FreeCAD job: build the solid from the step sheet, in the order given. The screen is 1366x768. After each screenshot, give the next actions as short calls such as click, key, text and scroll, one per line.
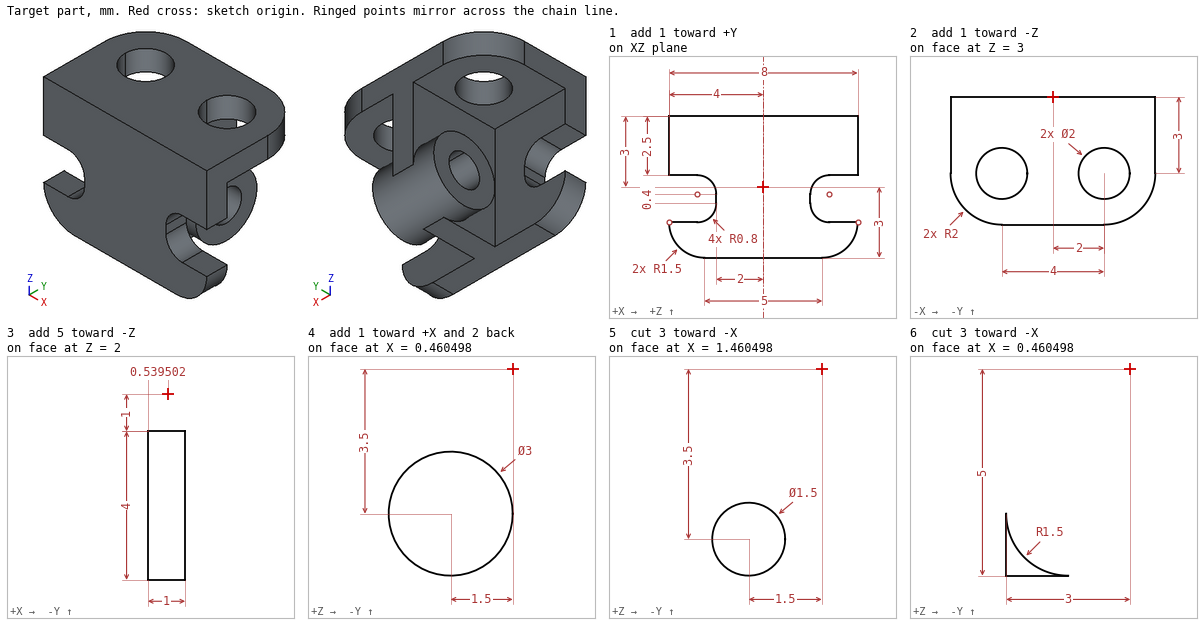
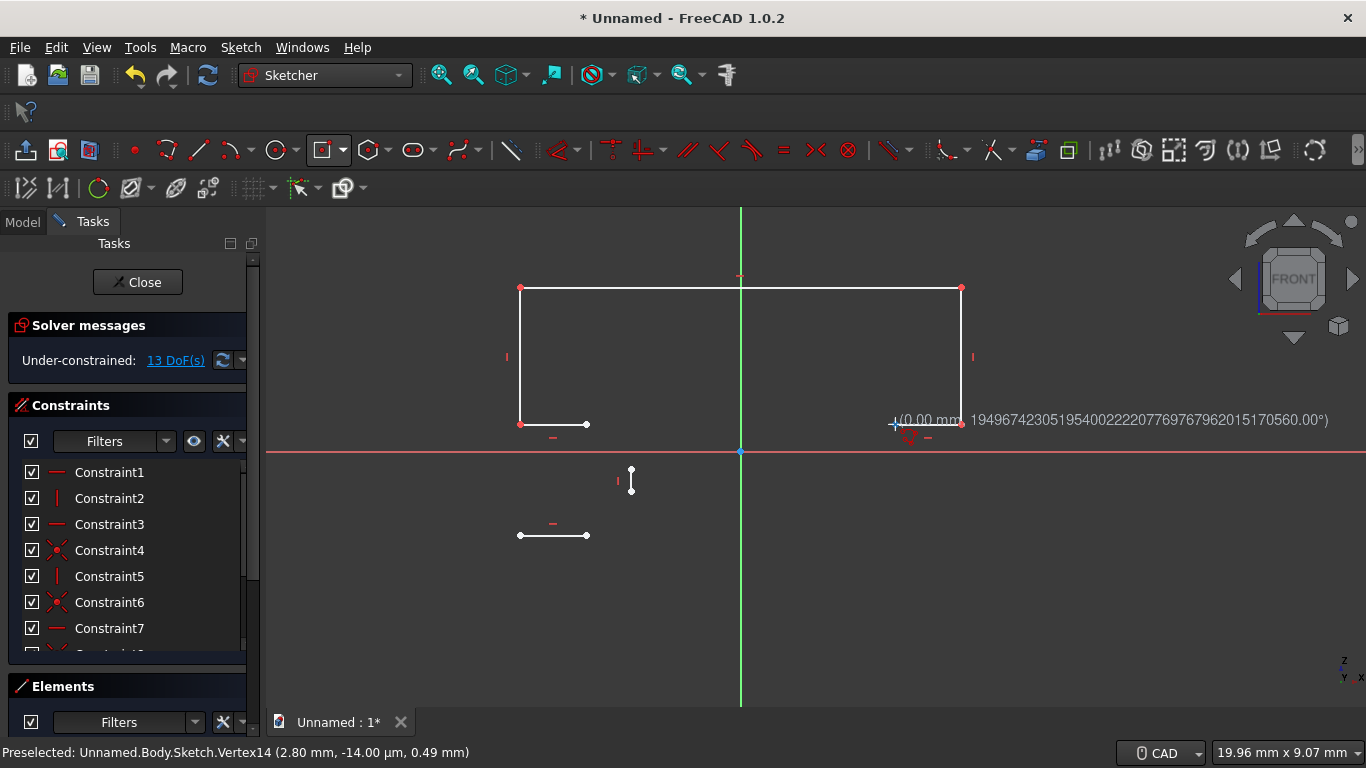
click(200, 150)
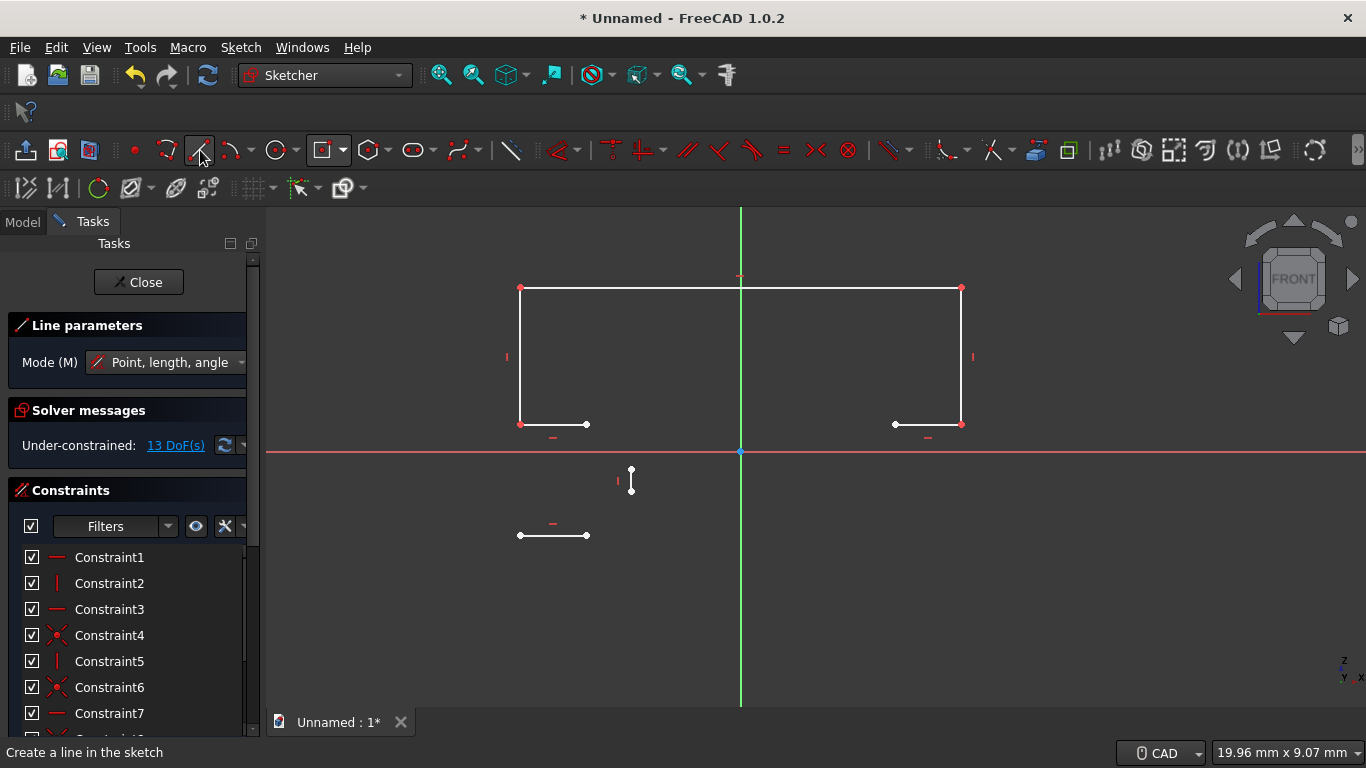
click(851, 469)
click(851, 491)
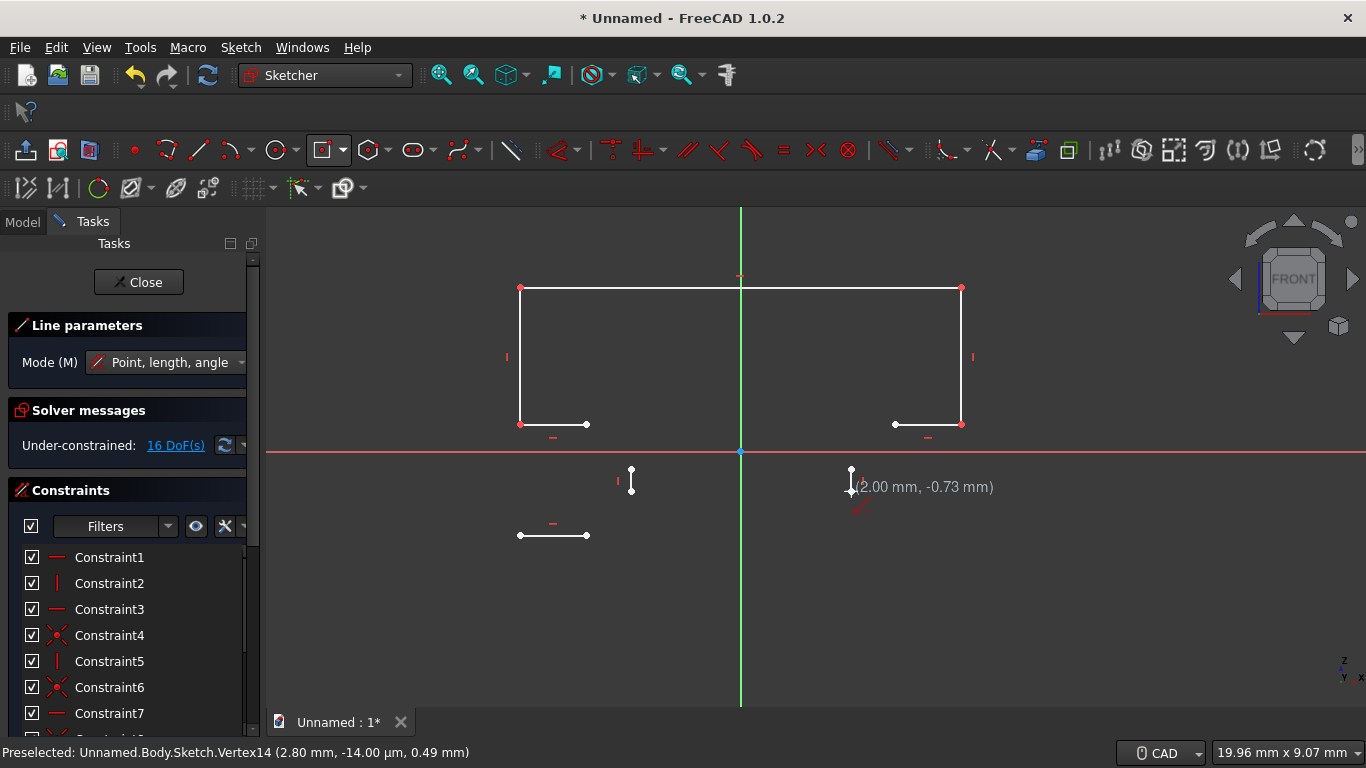
click(895, 535)
click(961, 535)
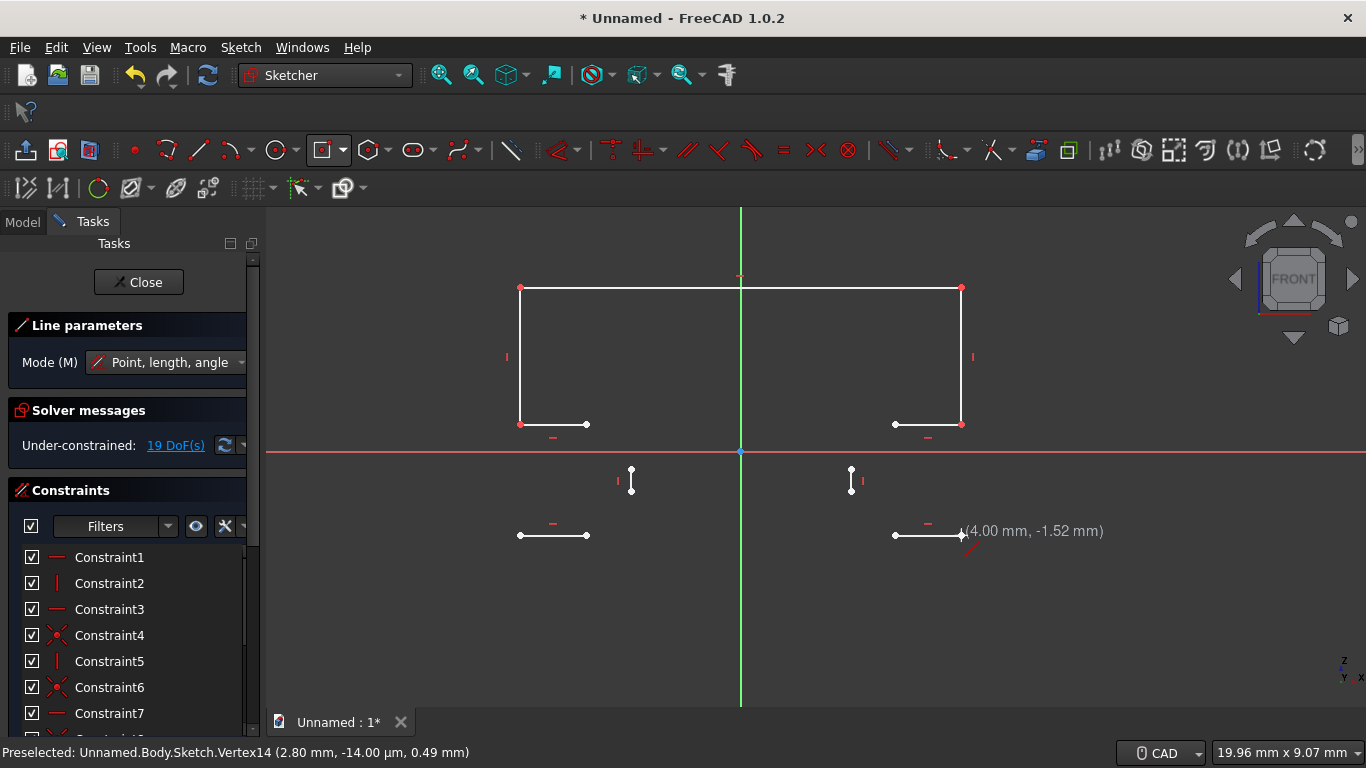
click(879, 617)
click(603, 617)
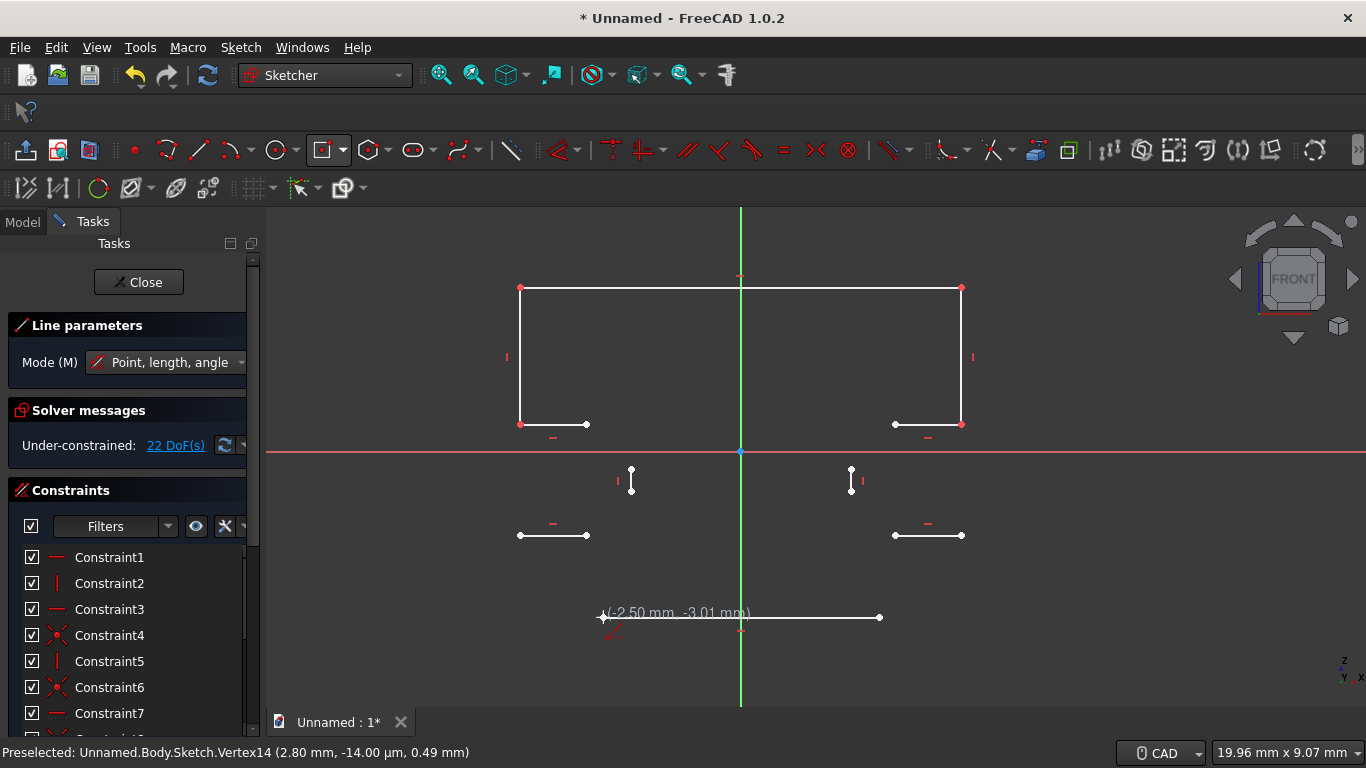
click(254, 150)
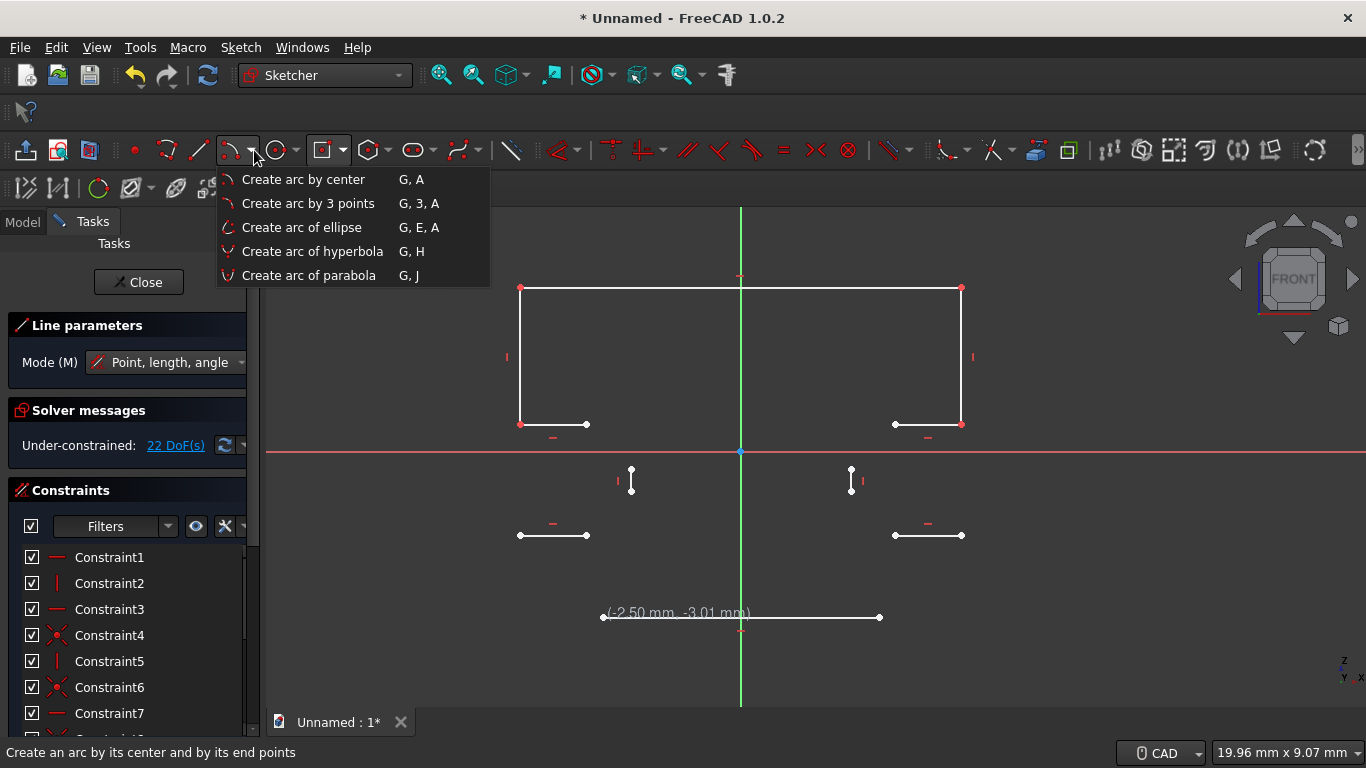
click(354, 203)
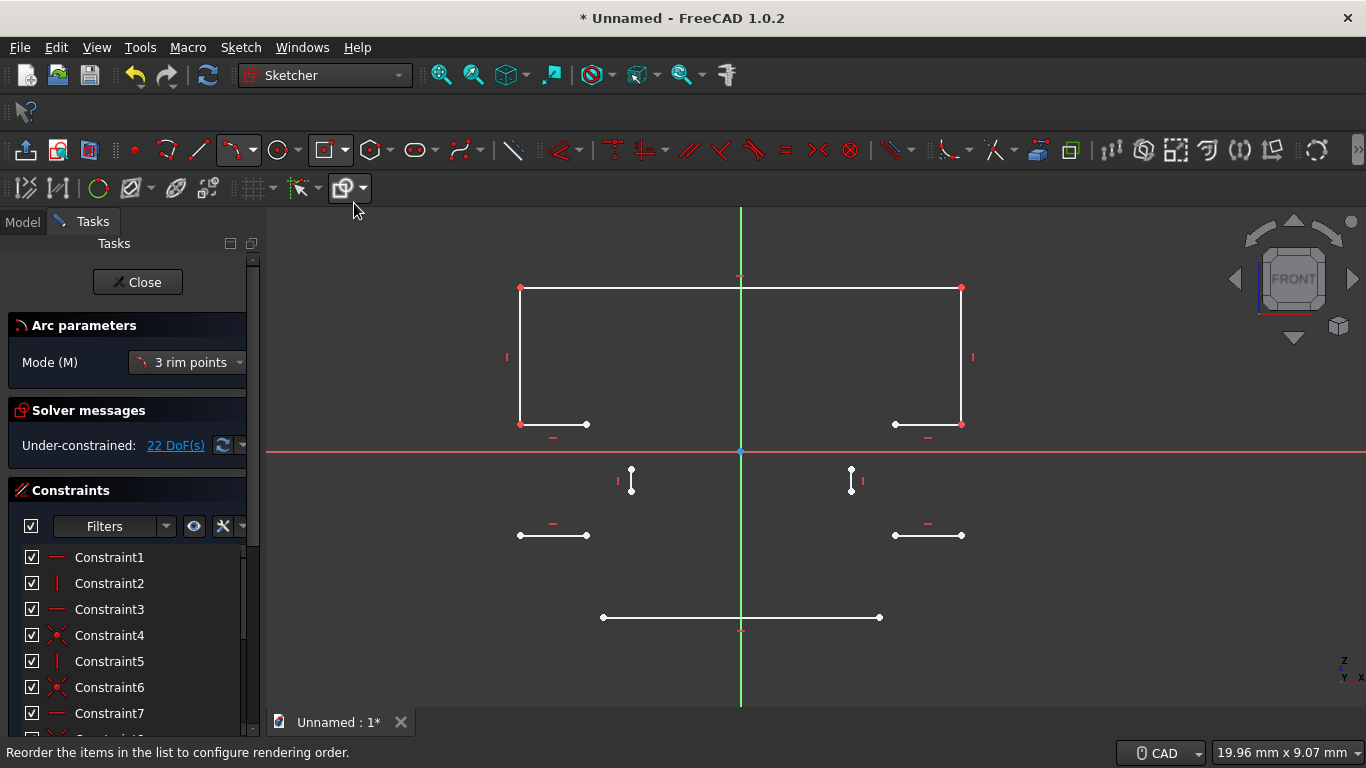
click(586, 536)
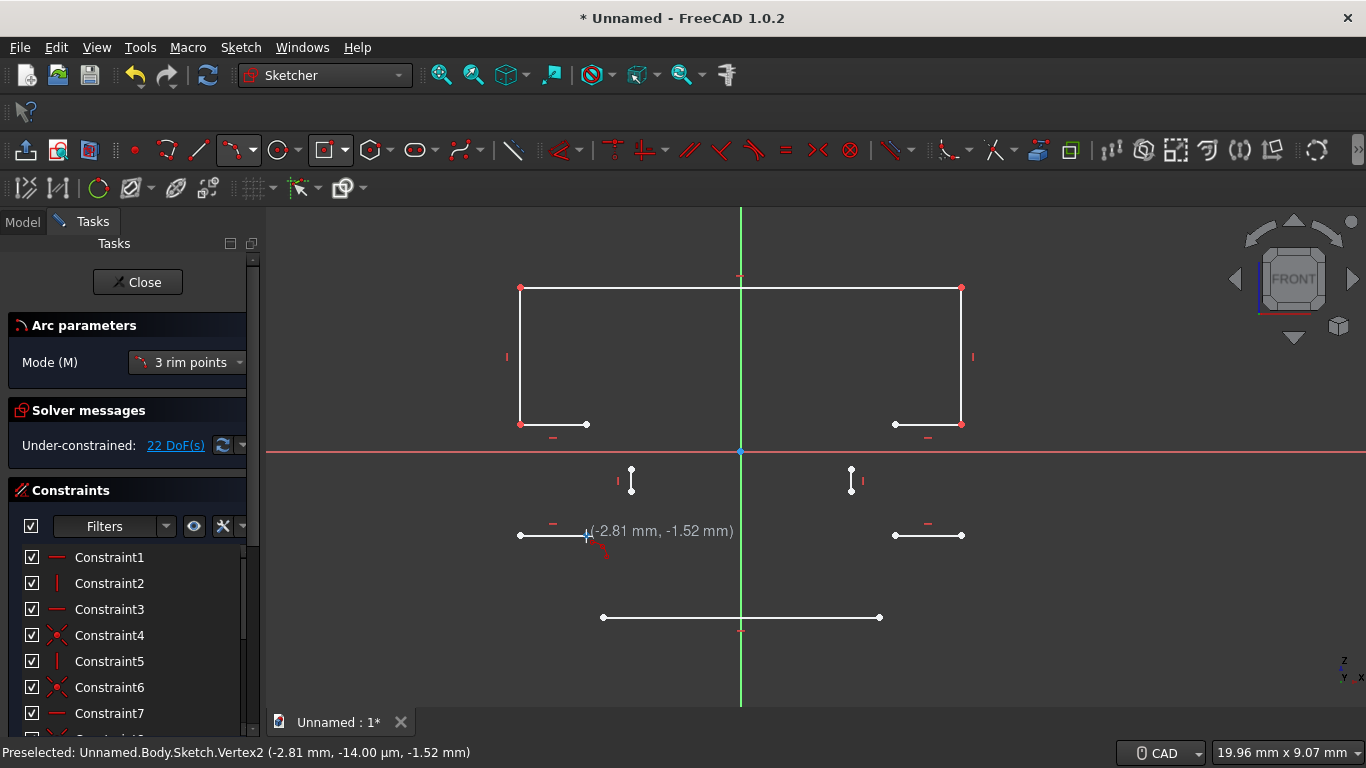
scroll(631, 491, up, 2)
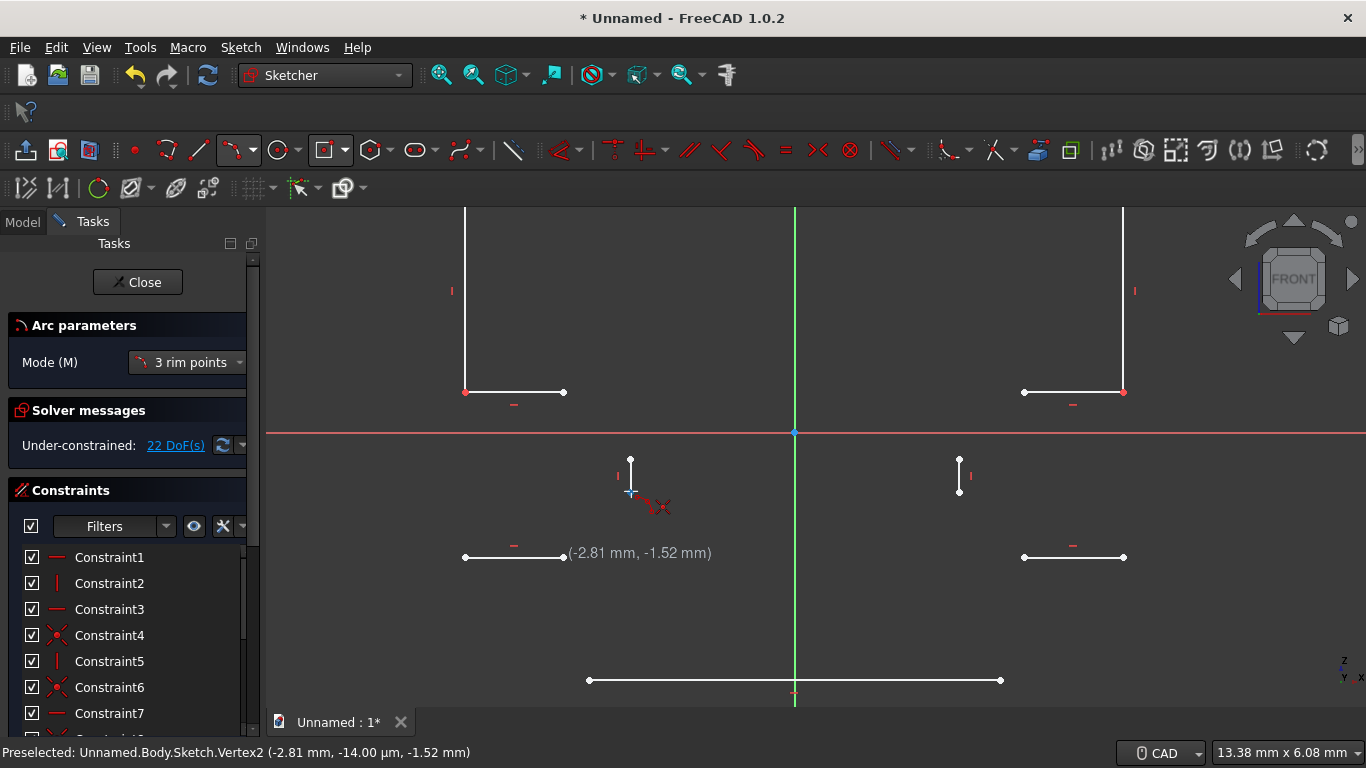
click(631, 492)
click(611, 537)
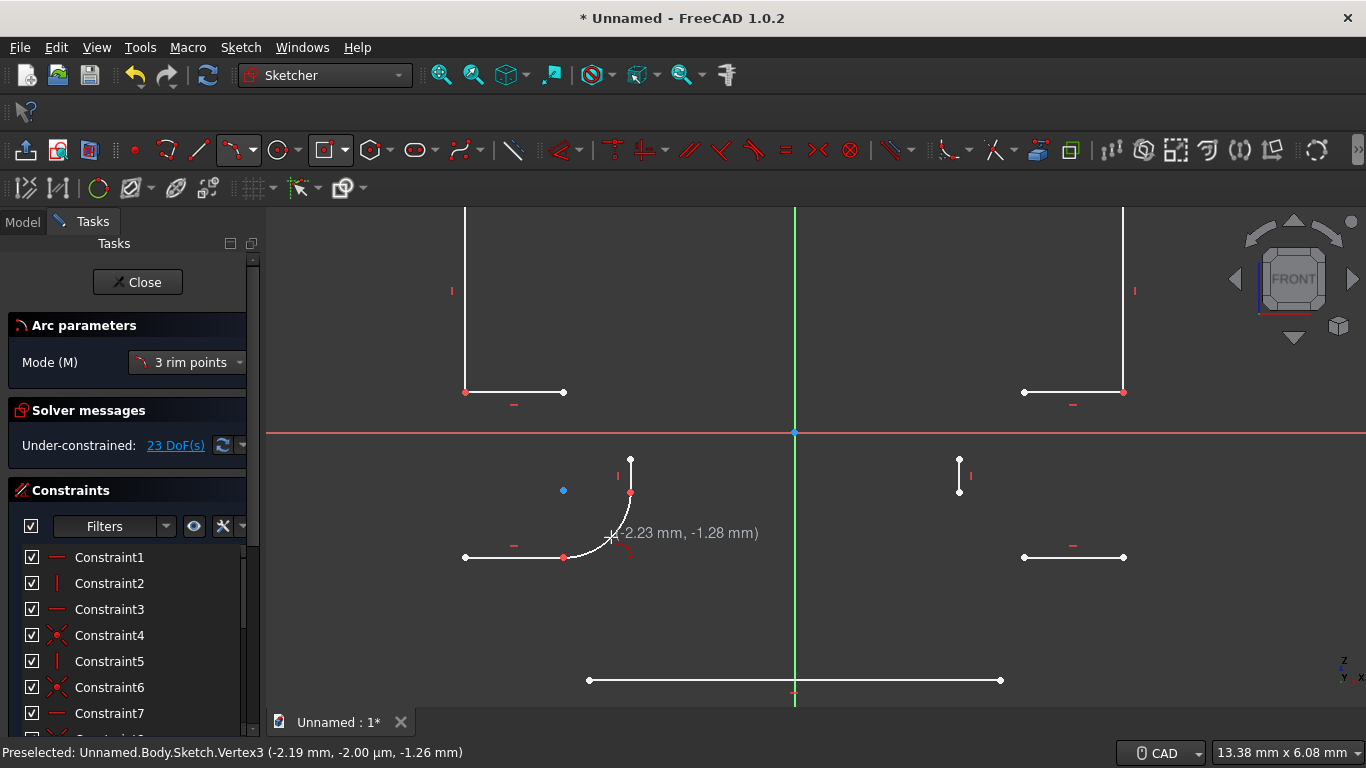
click(631, 459)
click(564, 392)
click(611, 411)